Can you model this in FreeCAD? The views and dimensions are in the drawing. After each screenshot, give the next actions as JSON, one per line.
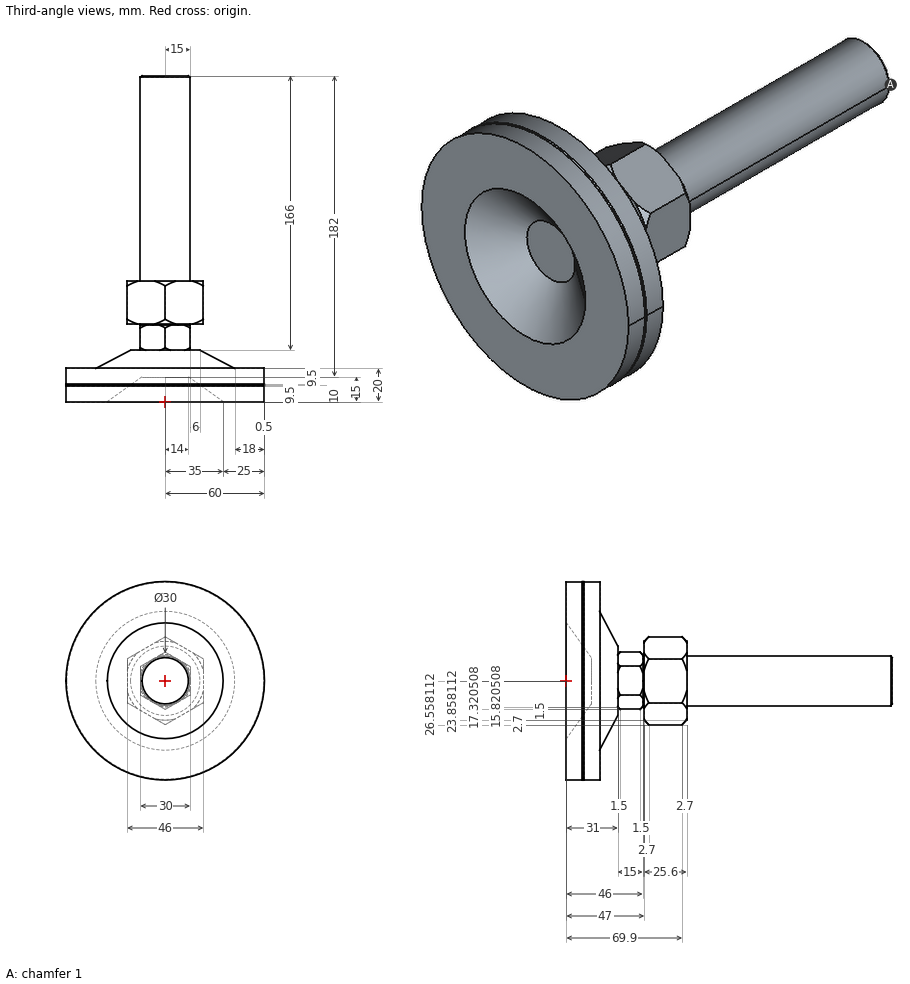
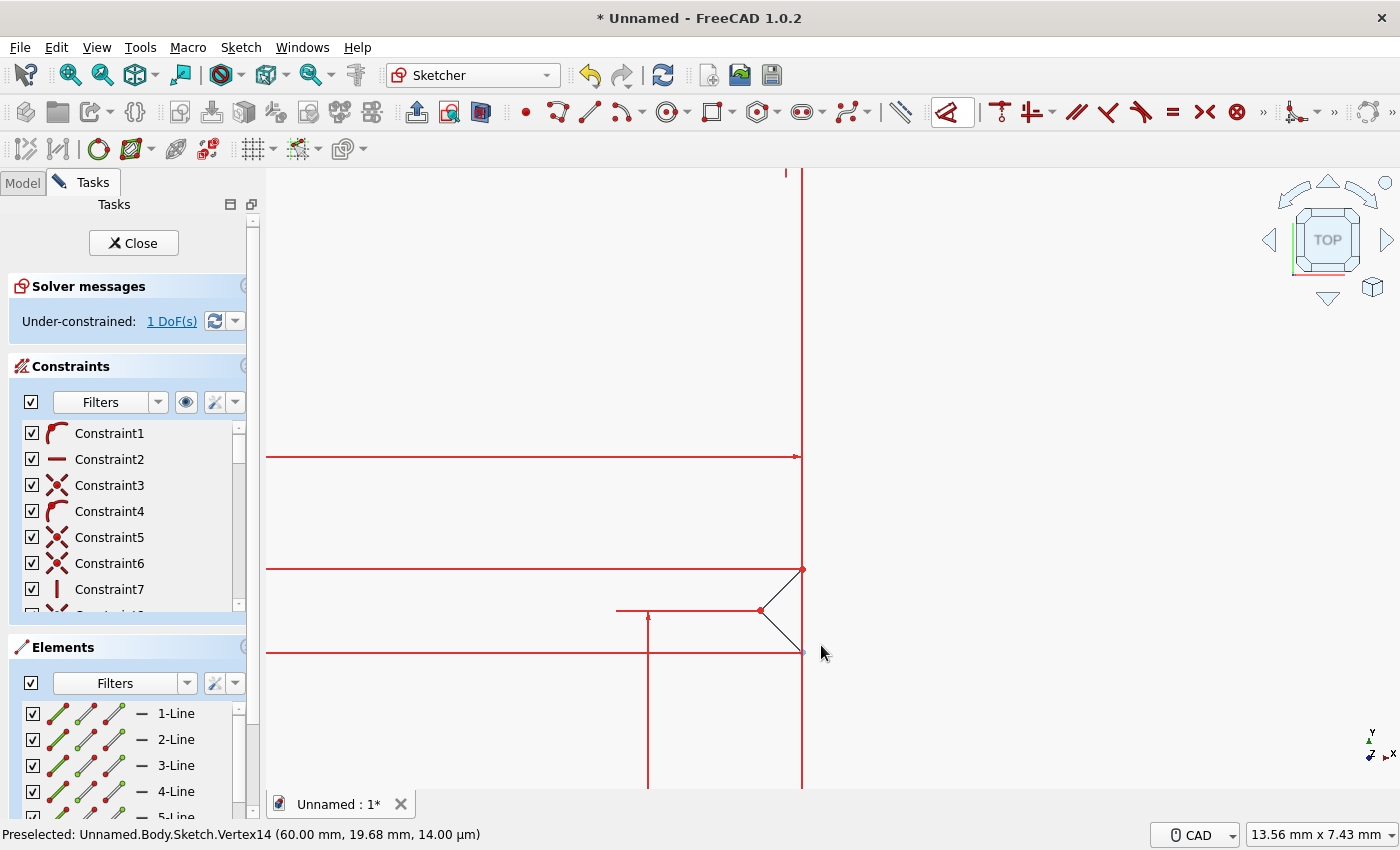
{"action": "left_click", "coordinate": [781, 632]}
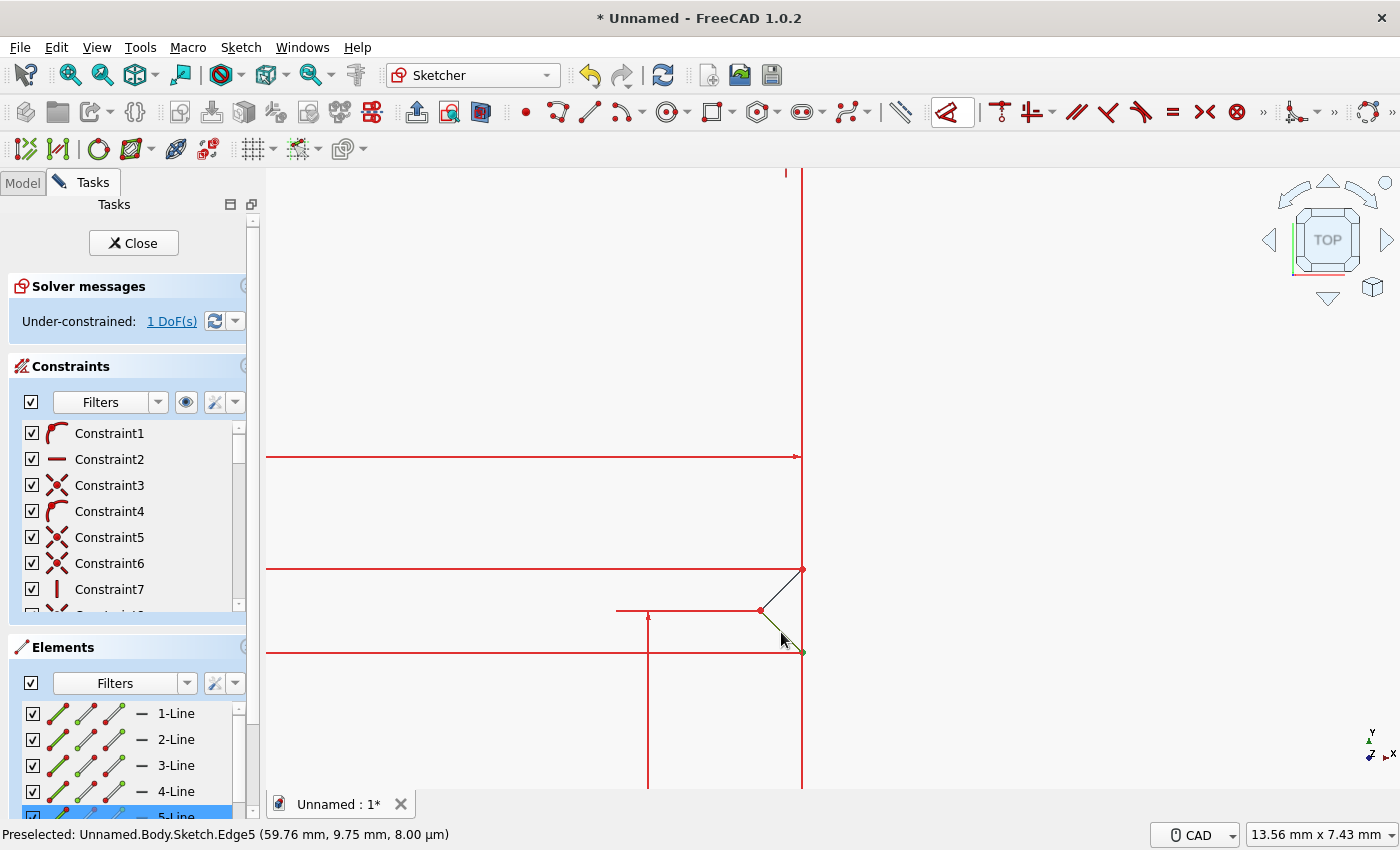
{"action": "key", "text": "l"}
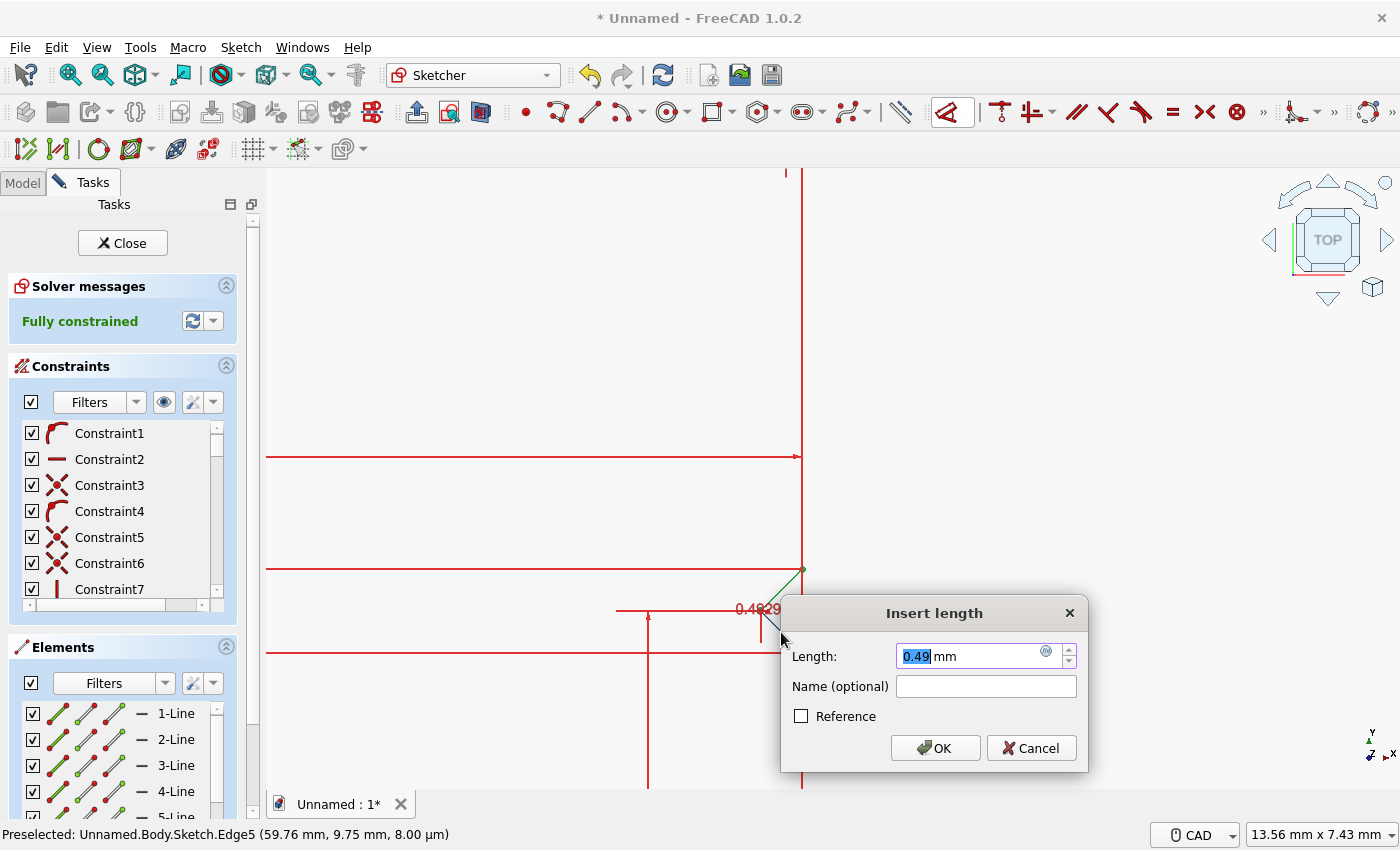
{"action": "type", "text": "0.5"}
{"action": "key", "text": "Return"}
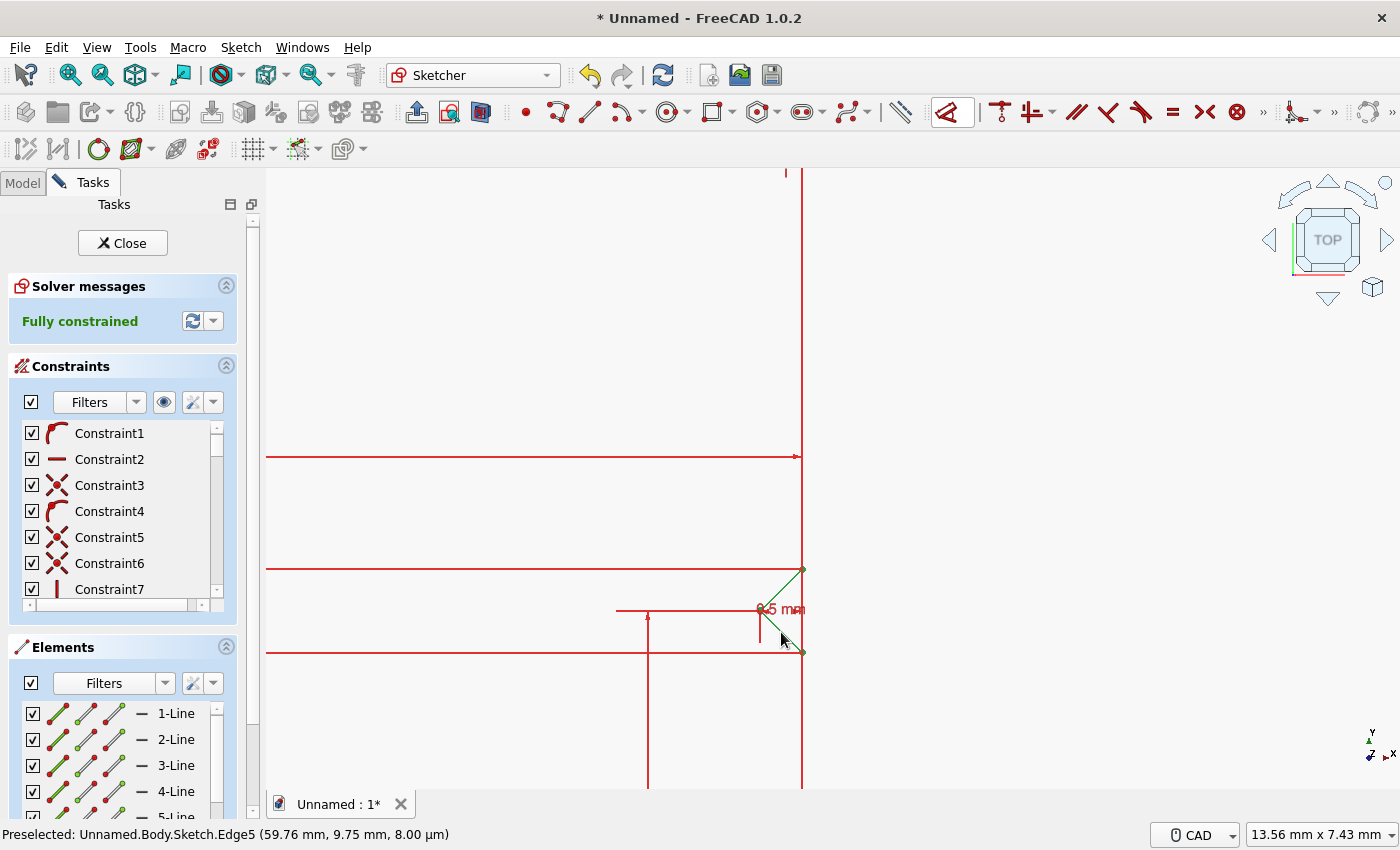
{"action": "left_click", "coordinate": [123, 243]}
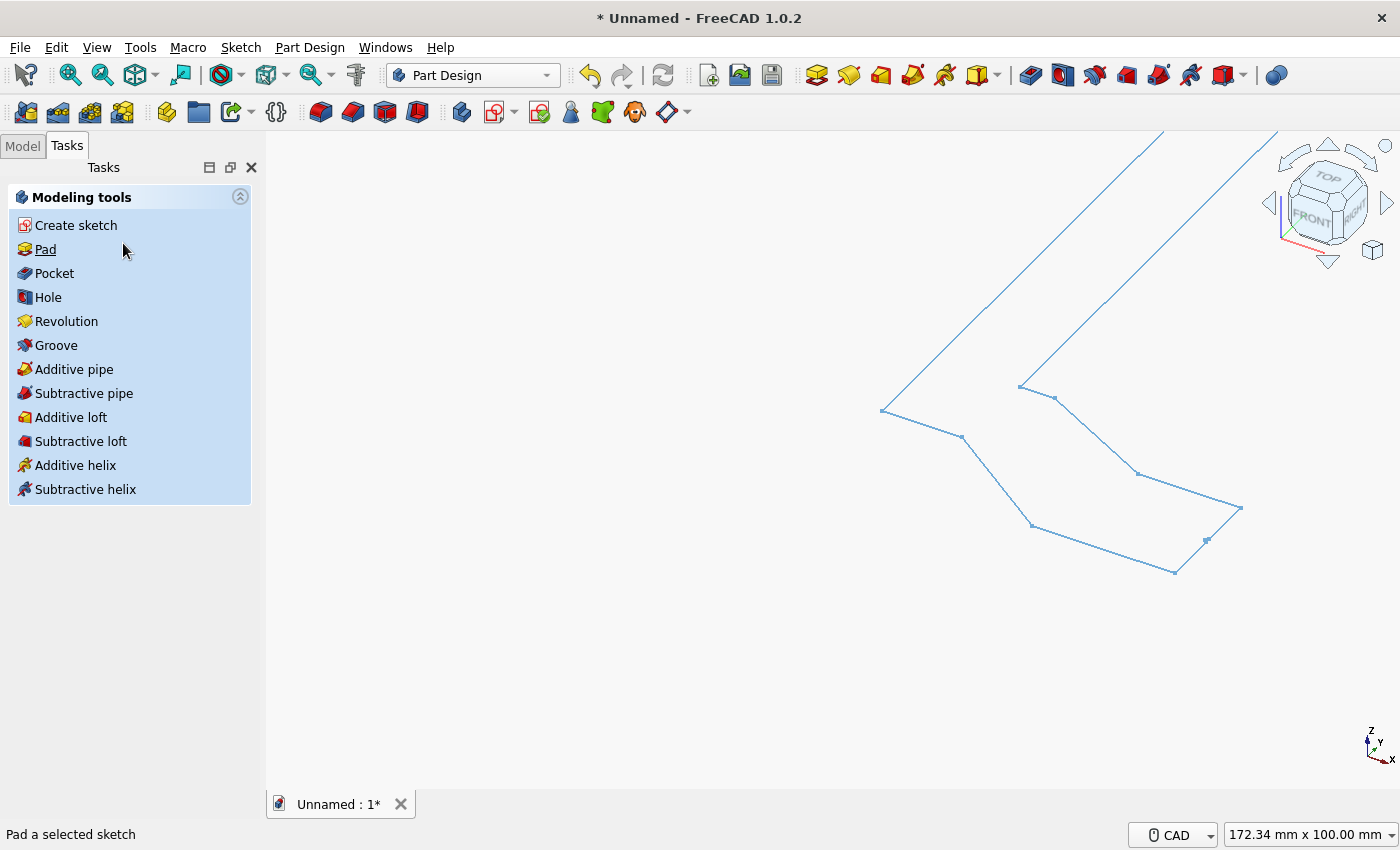
{"action": "left_click", "coordinate": [850, 76]}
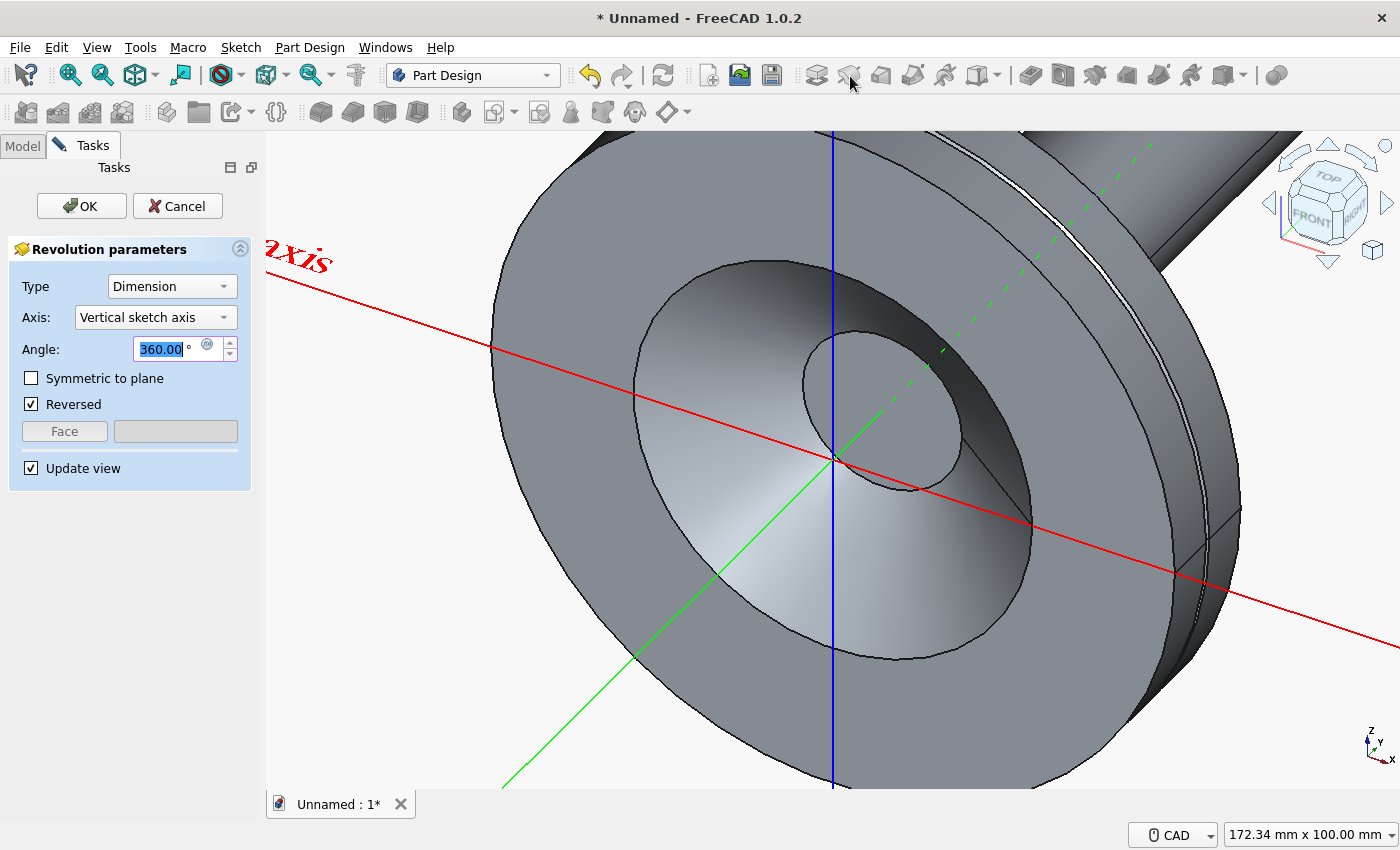
{"action": "left_click", "coordinate": [82, 206]}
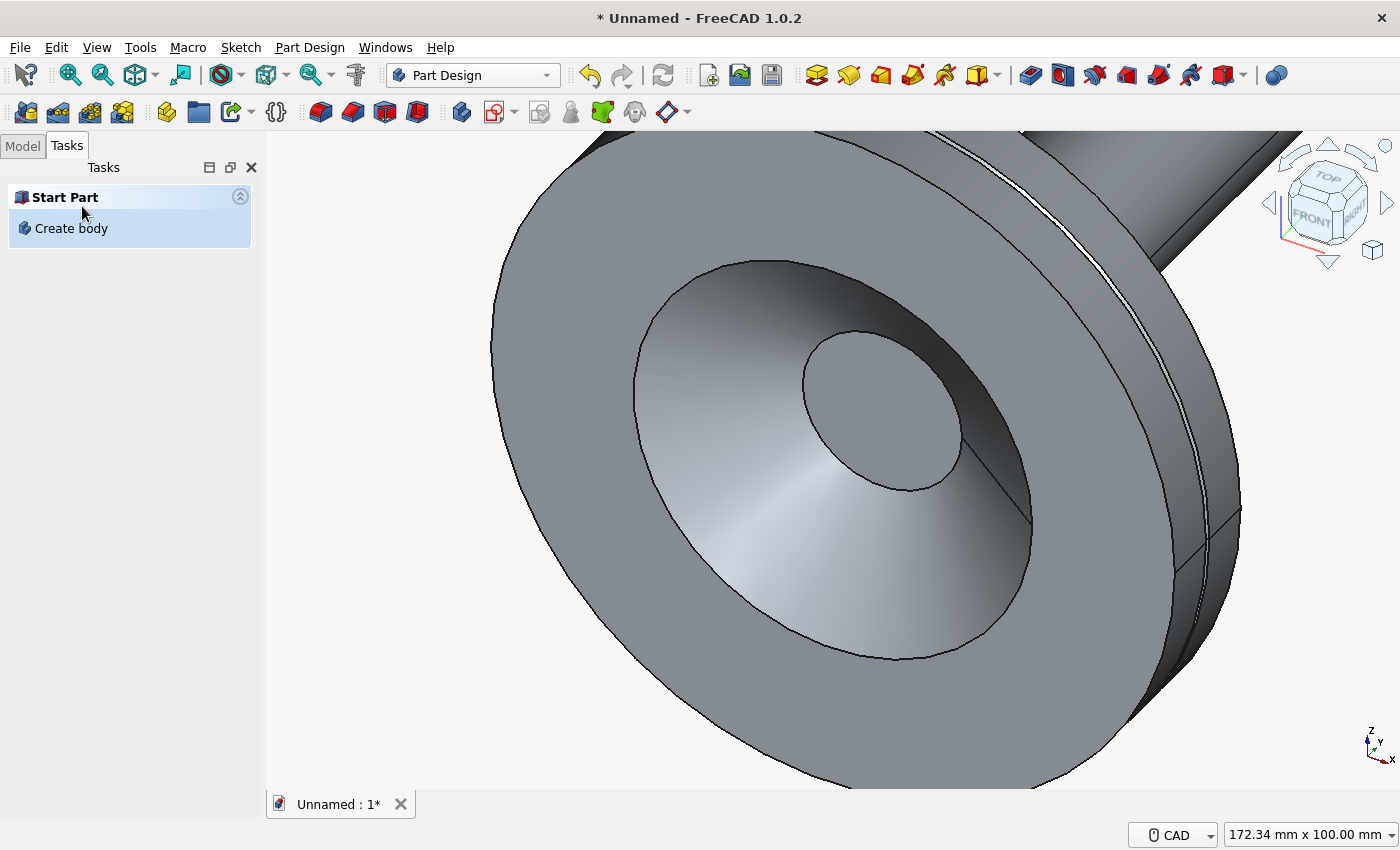
{"action": "key", "text": "v f"}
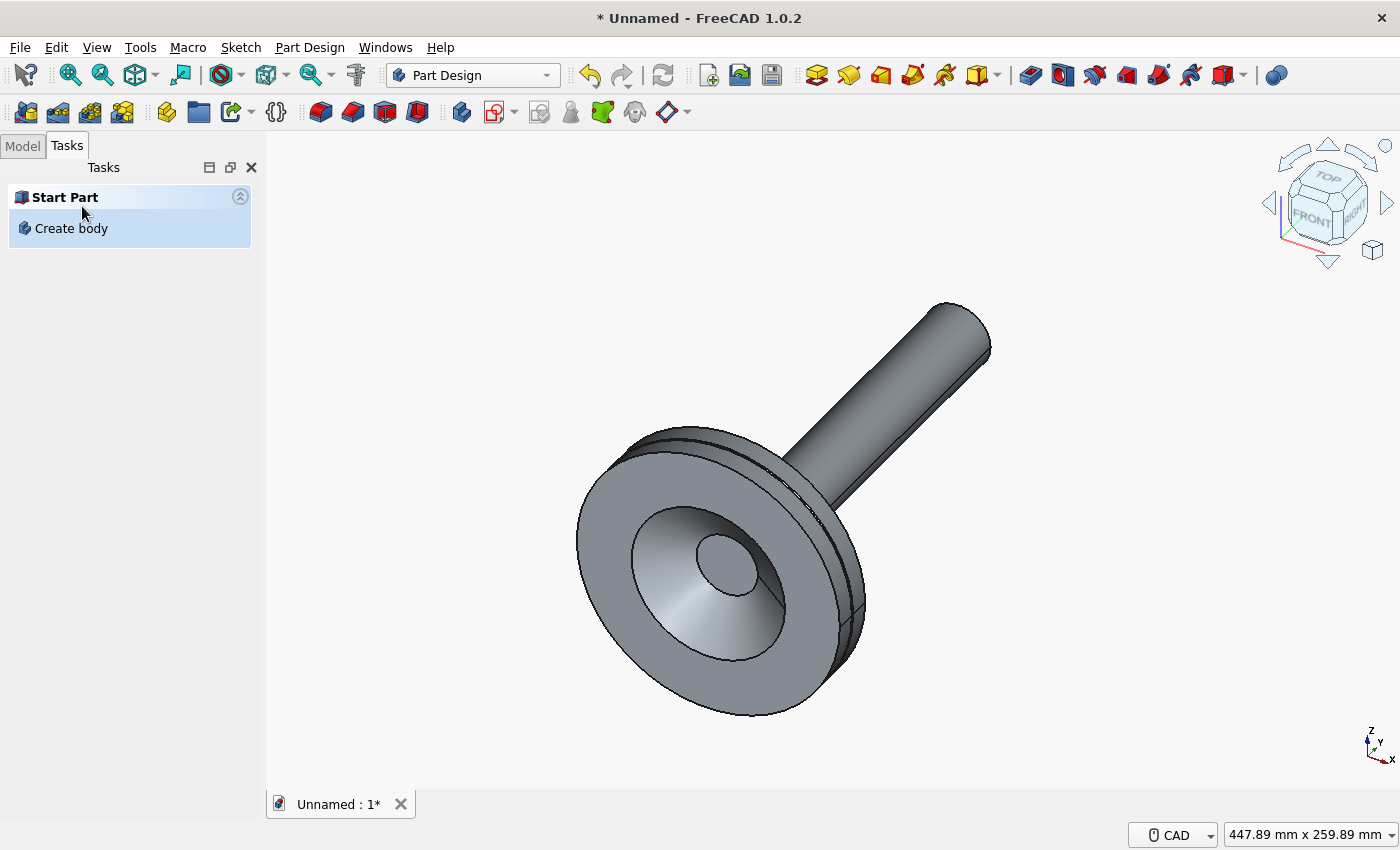
{"action": "key", "text": "4"}